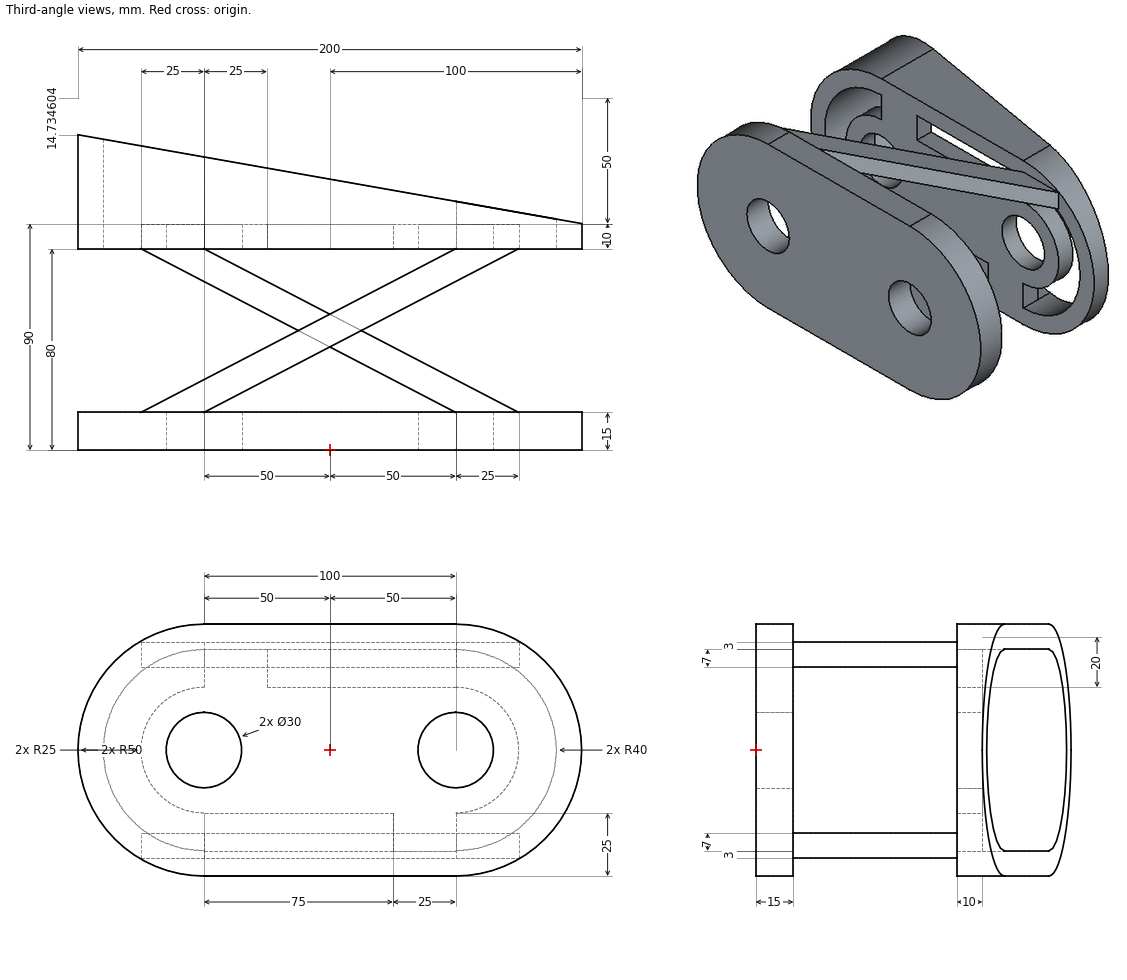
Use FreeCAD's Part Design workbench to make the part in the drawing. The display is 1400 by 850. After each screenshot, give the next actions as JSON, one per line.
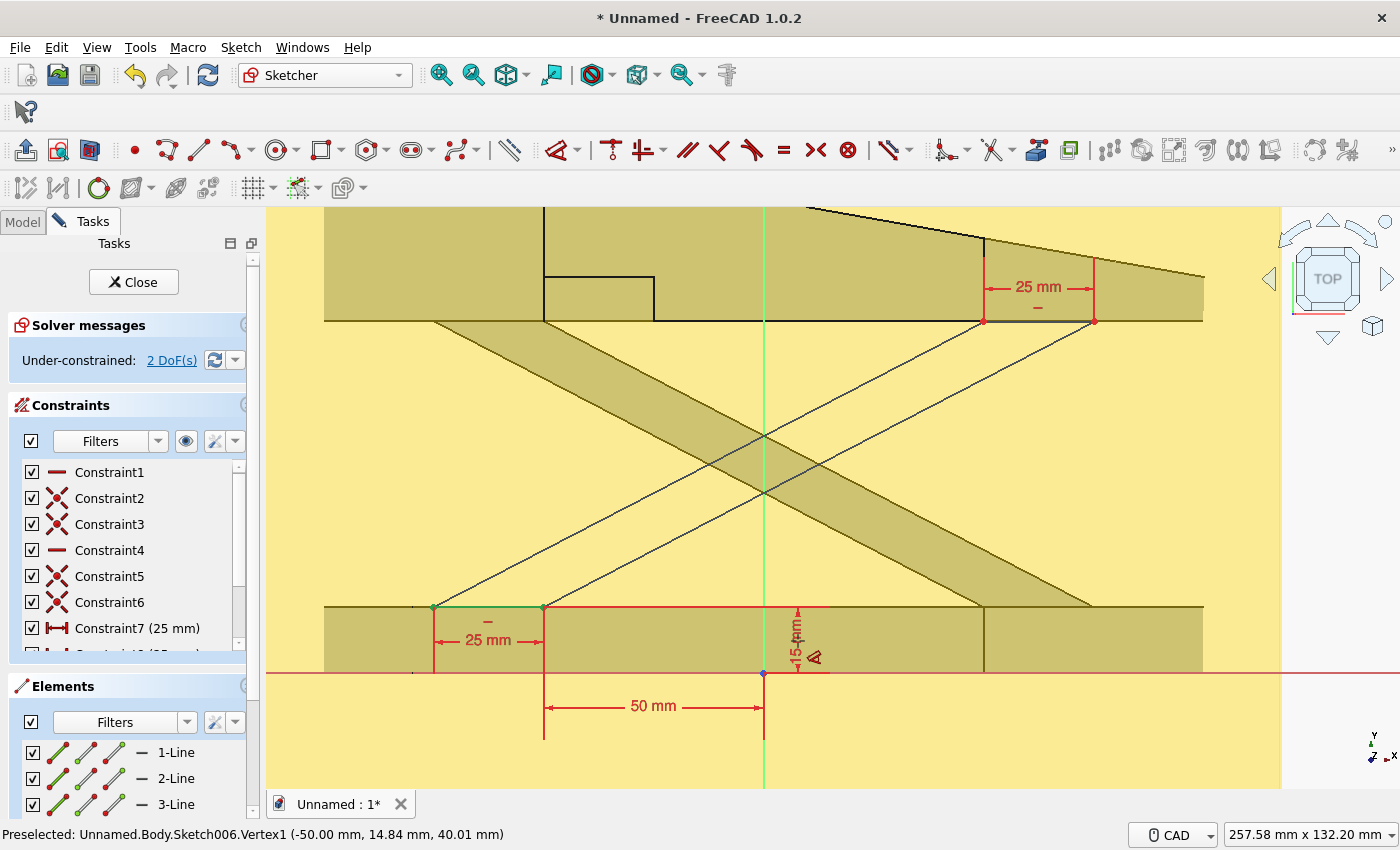
{"action": "left_click", "coordinate": [984, 322]}
{"action": "left_click", "coordinate": [874, 707]}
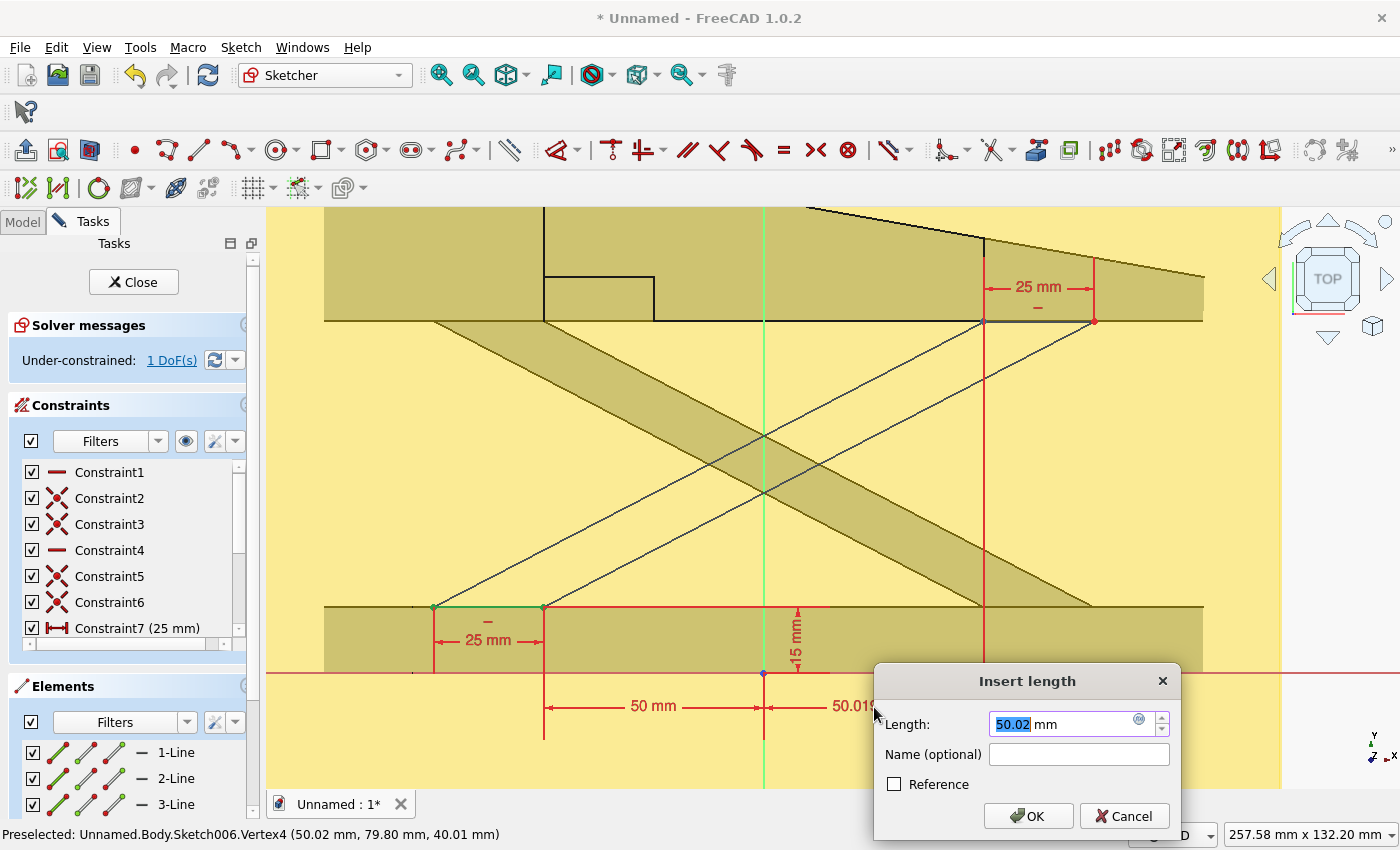
{"action": "type", "text": "50"}
{"action": "key", "text": "Return"}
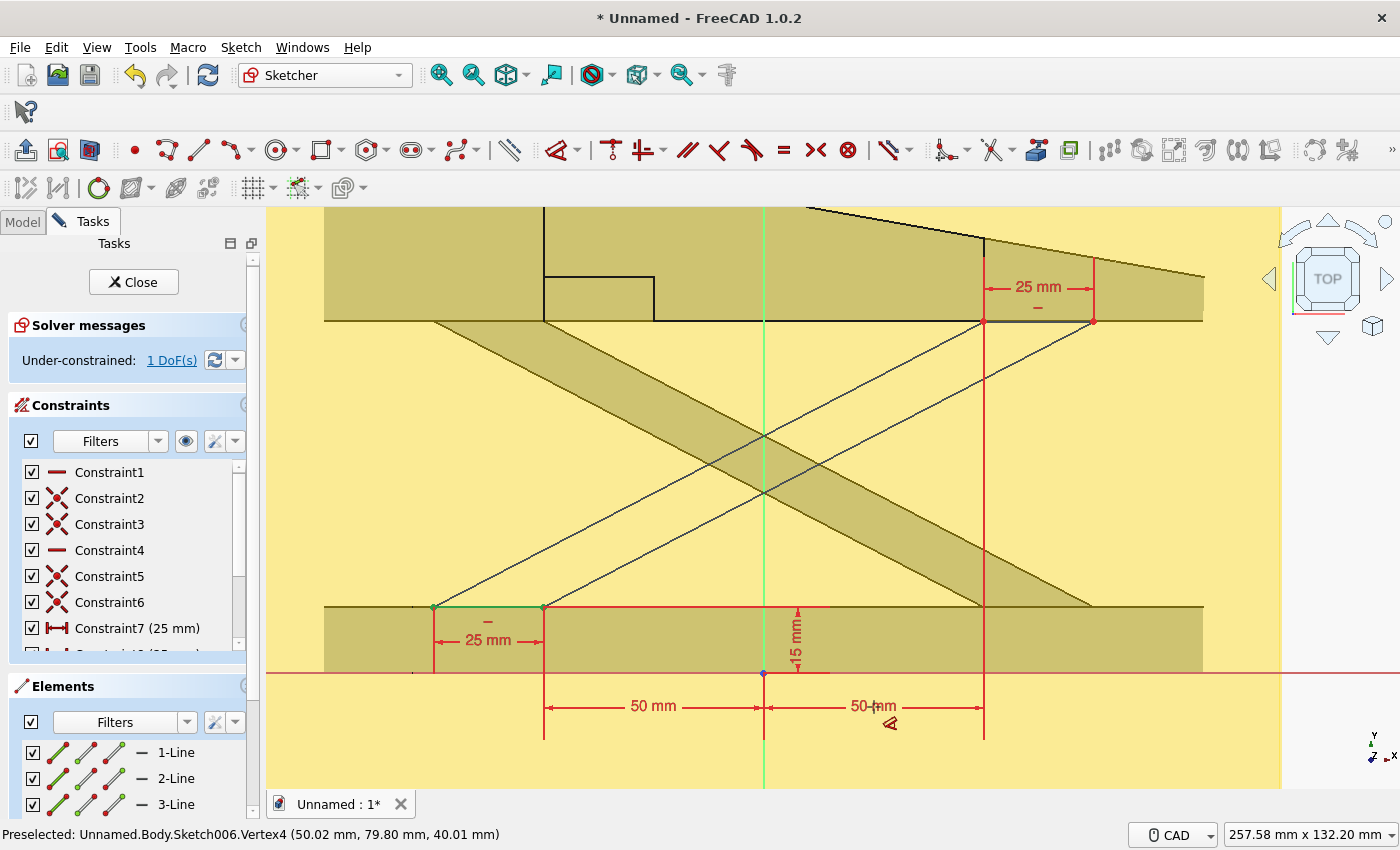
{"action": "left_click", "coordinate": [984, 322]}
{"action": "left_click", "coordinate": [1018, 498]}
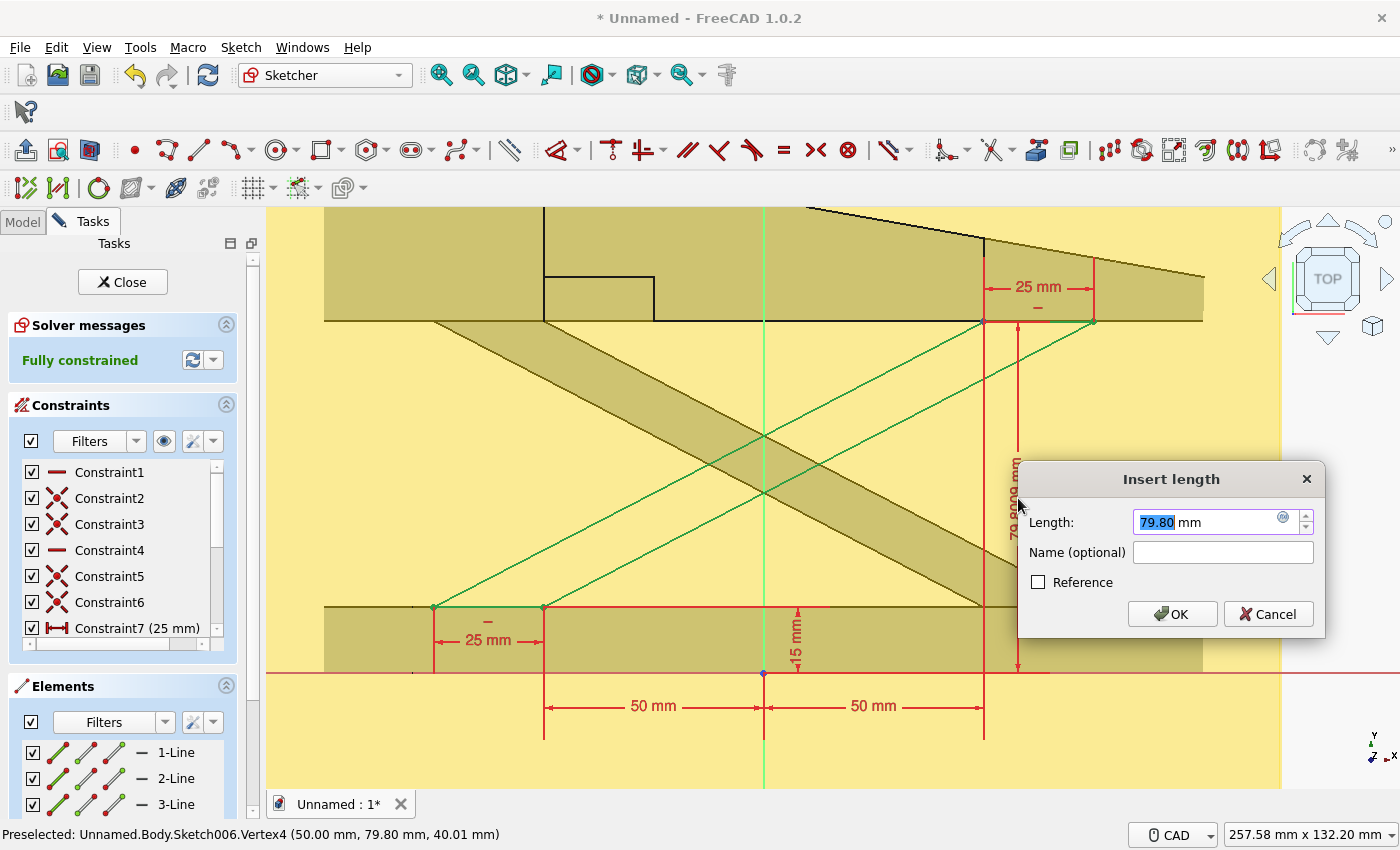
{"action": "type", "text": "80"}
{"action": "key", "text": "Return"}
{"action": "key", "text": "Escape"}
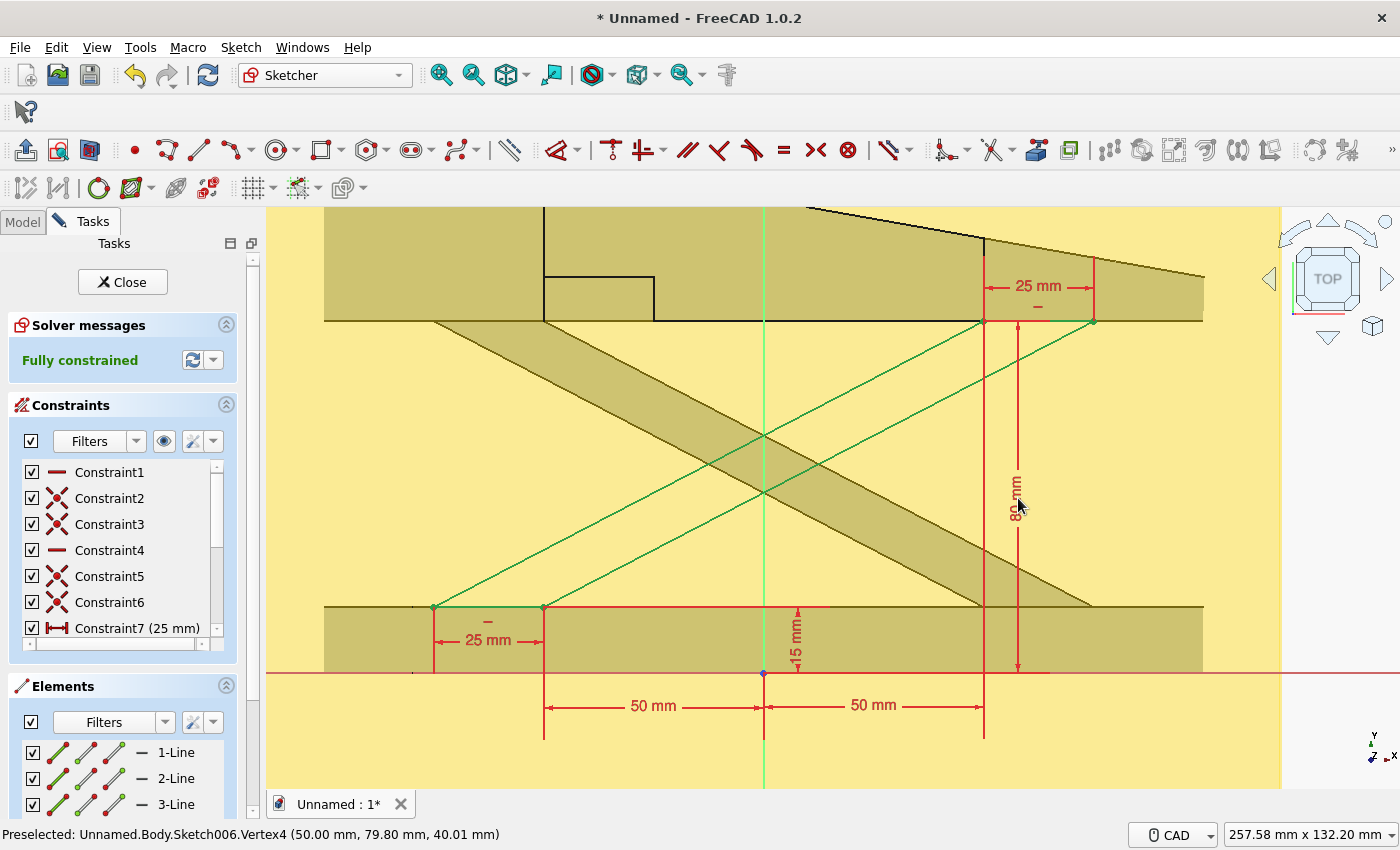
{"action": "left_click", "coordinate": [123, 282]}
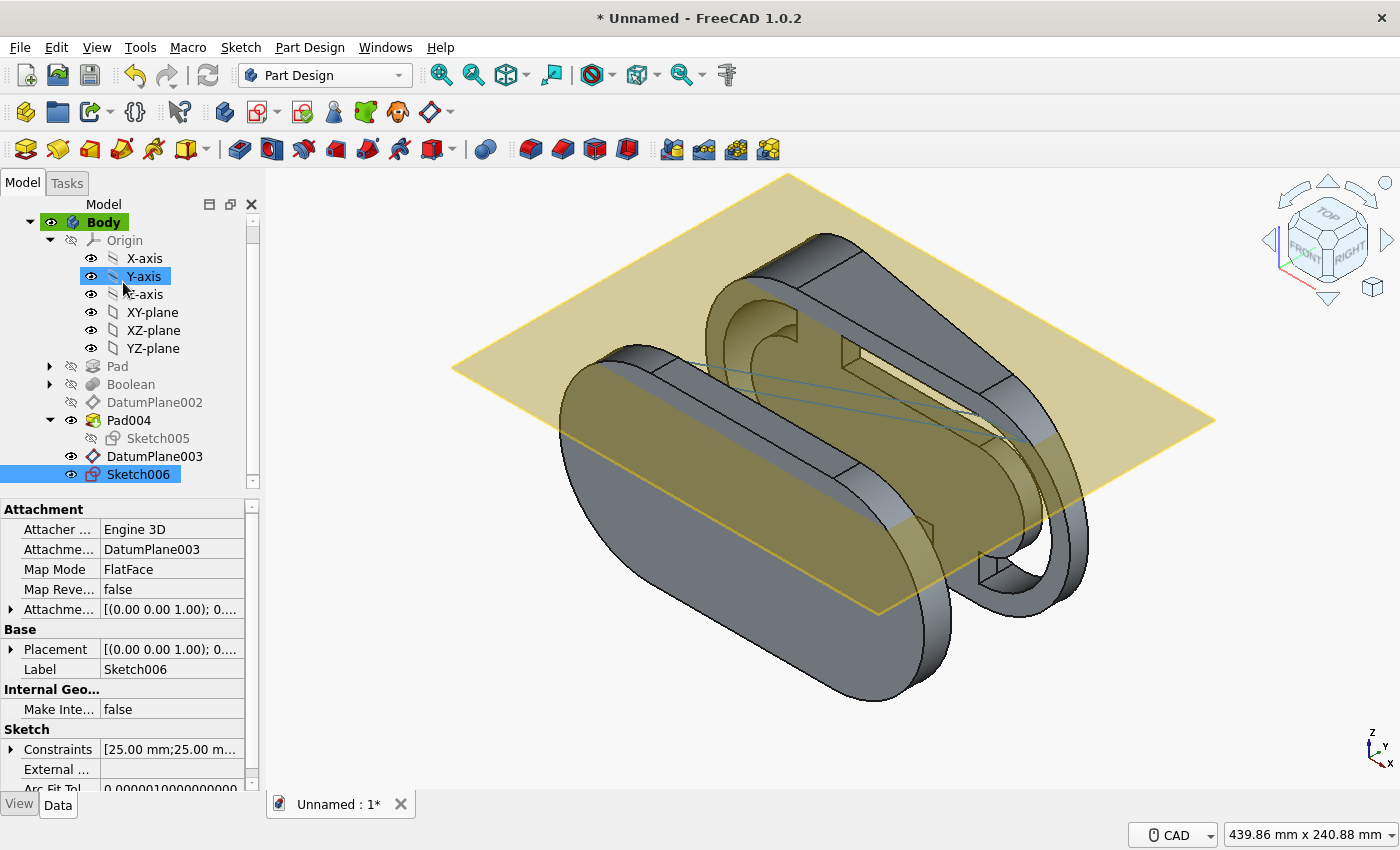
{"action": "left_click", "coordinate": [26, 150]}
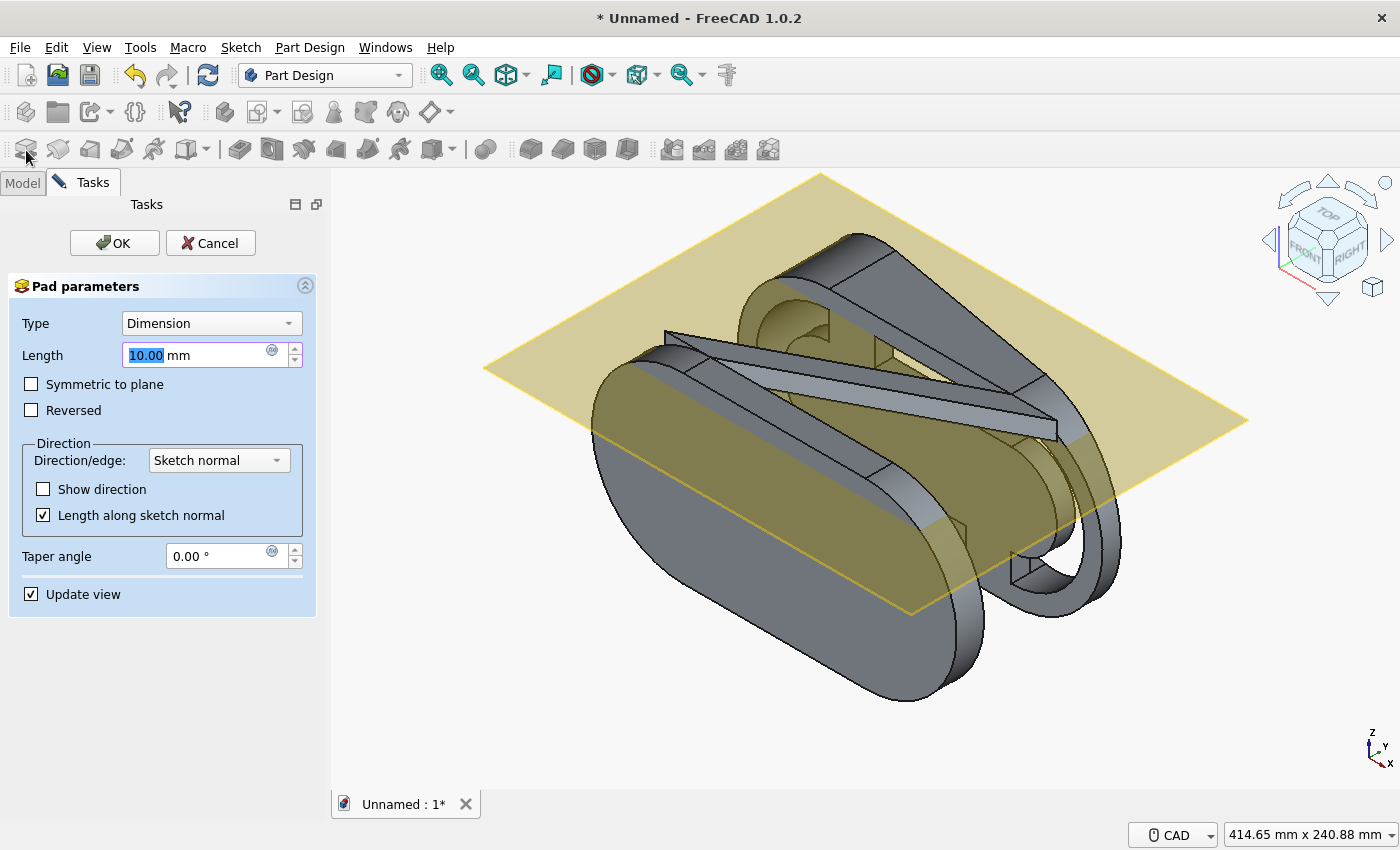
{"action": "left_click", "coordinate": [212, 324]}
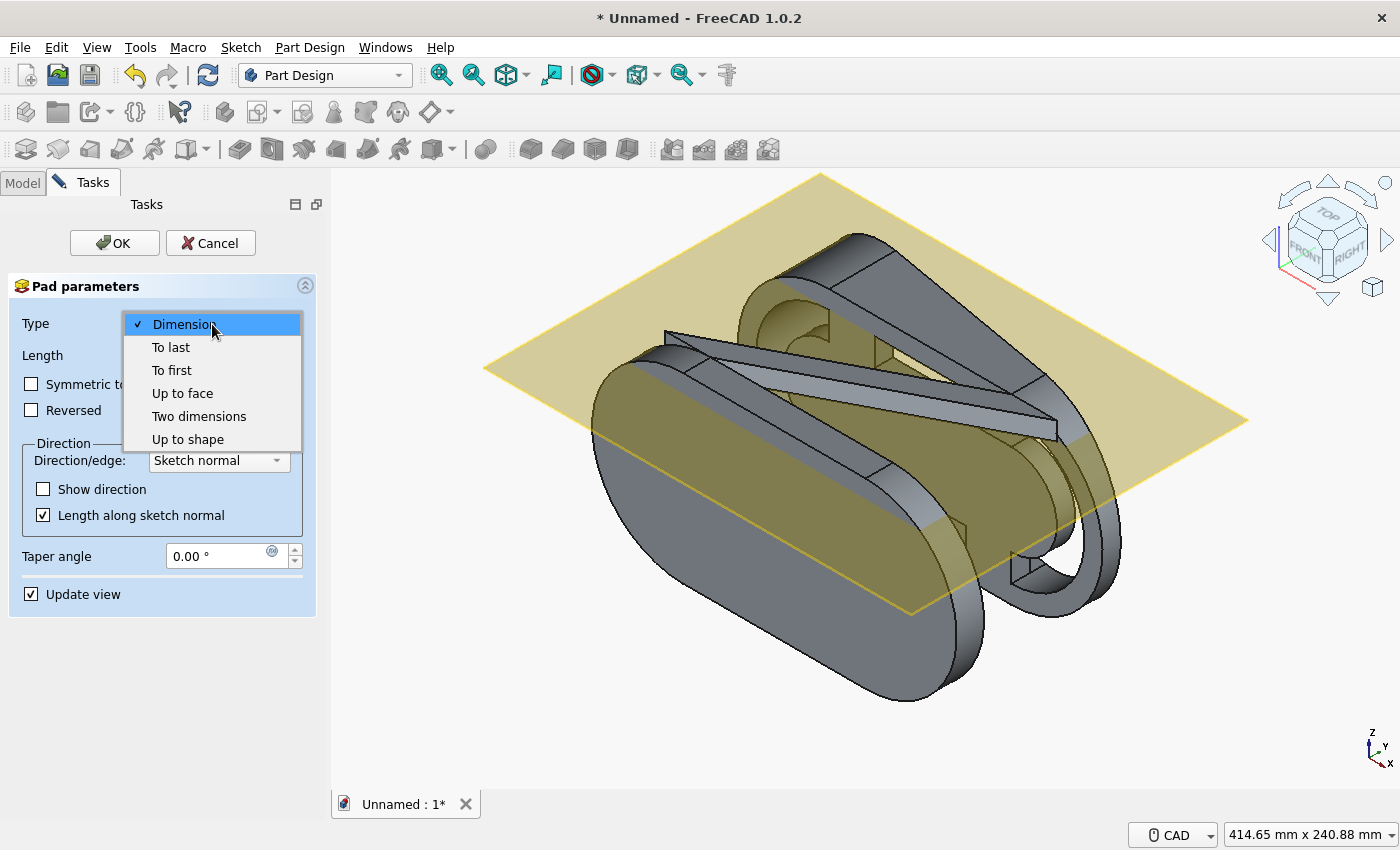
{"action": "left_click", "coordinate": [212, 416]}